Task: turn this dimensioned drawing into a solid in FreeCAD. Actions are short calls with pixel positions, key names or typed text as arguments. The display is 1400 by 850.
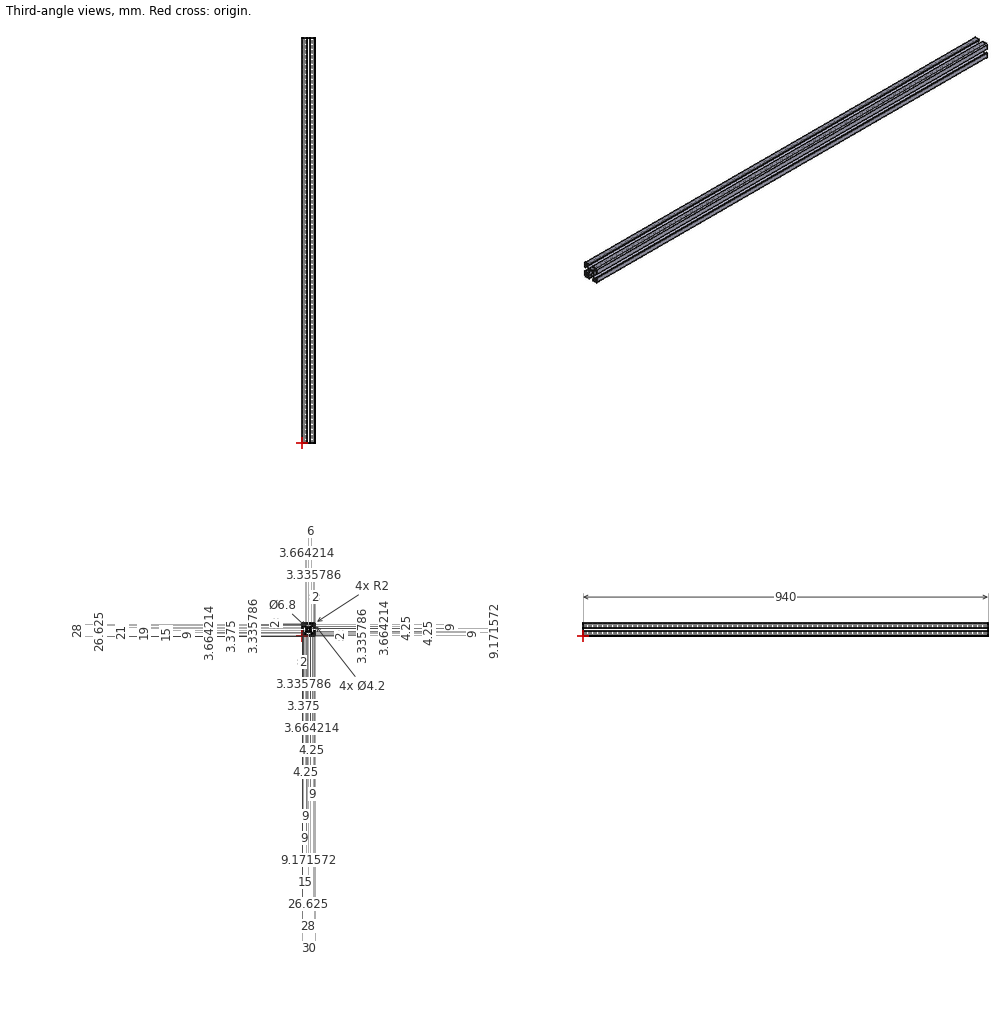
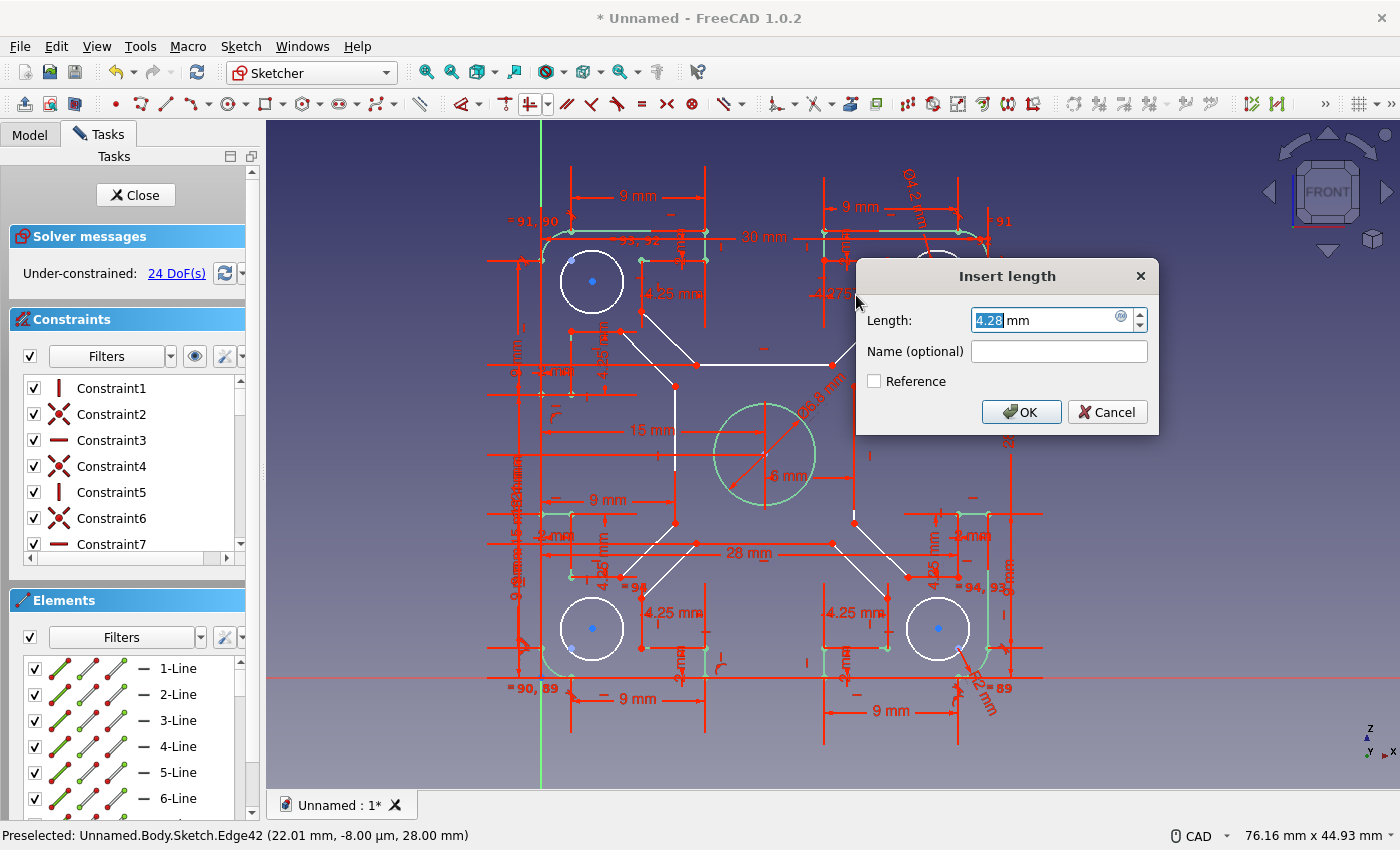
text(4.25)
key(Return)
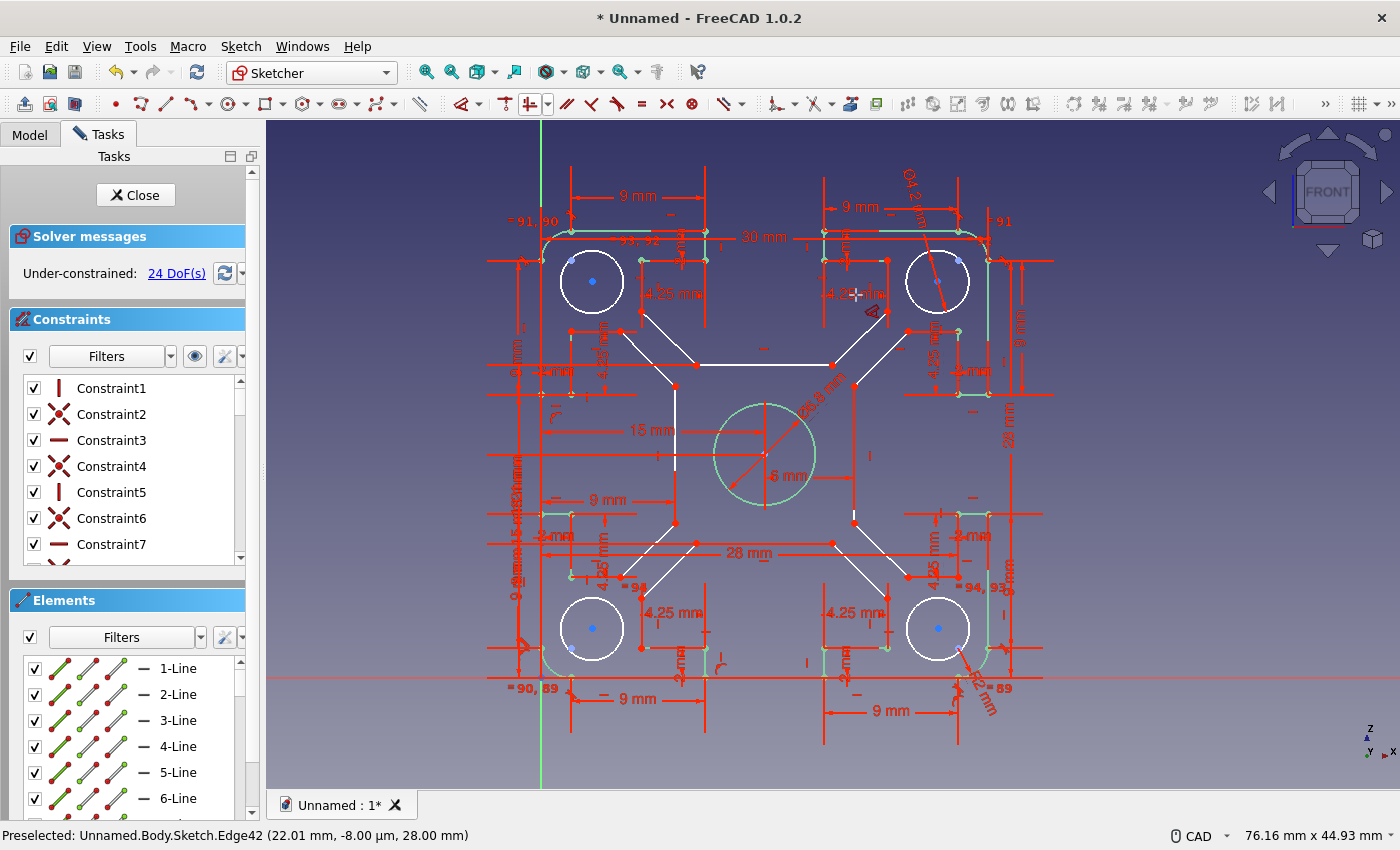
click(592, 282)
click(567, 712)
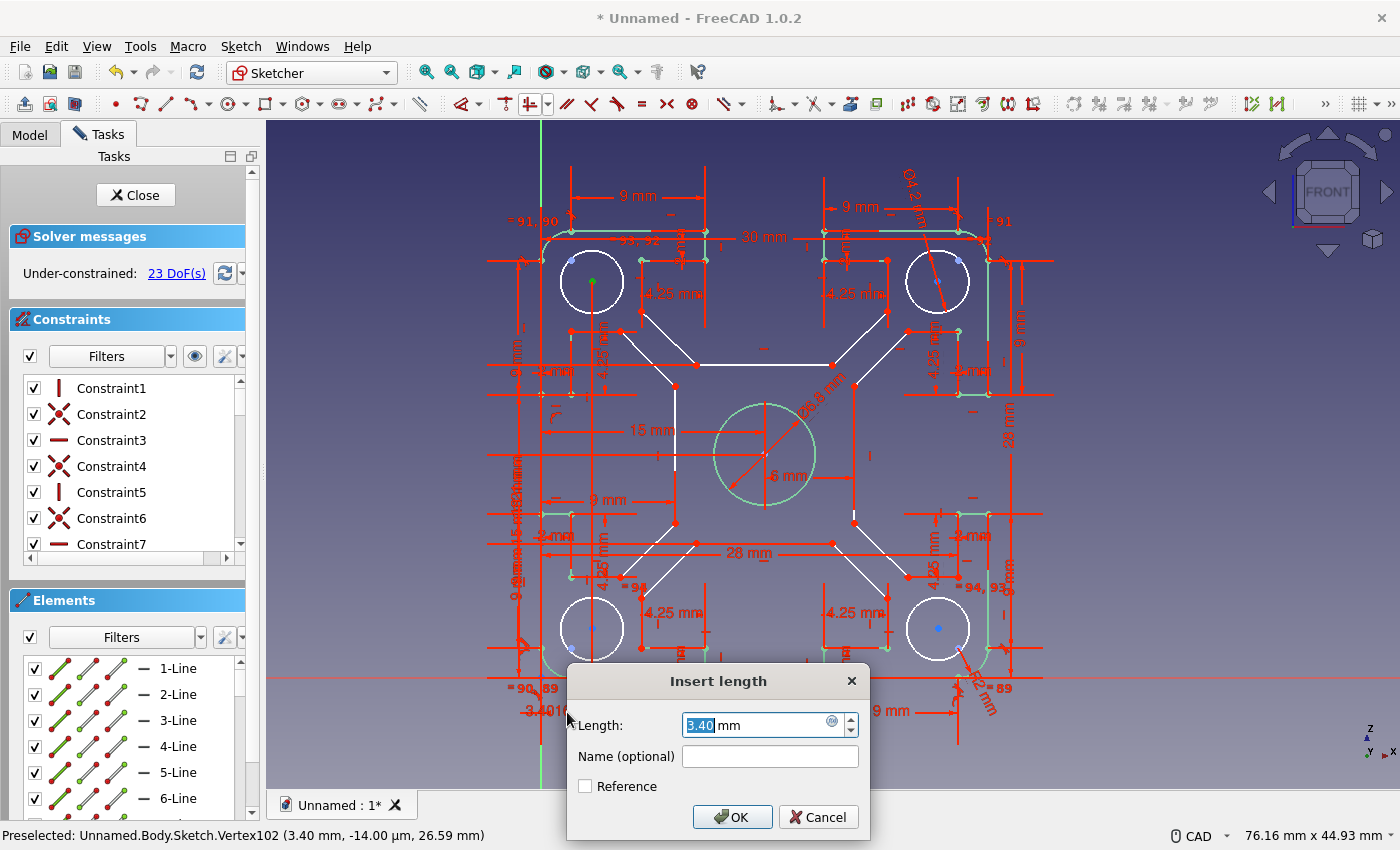
text(3.375)
key(Return)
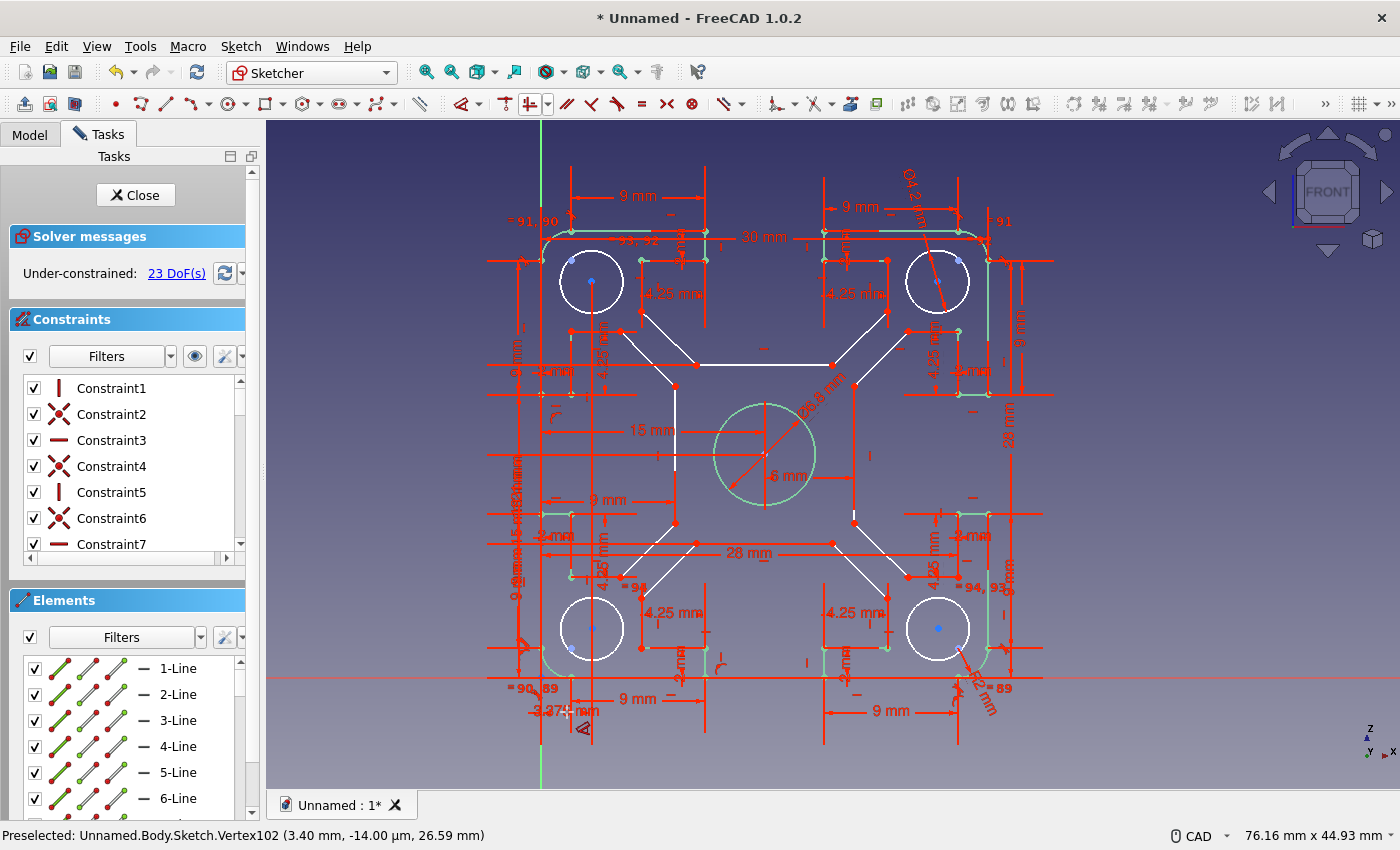
click(938, 629)
click(507, 653)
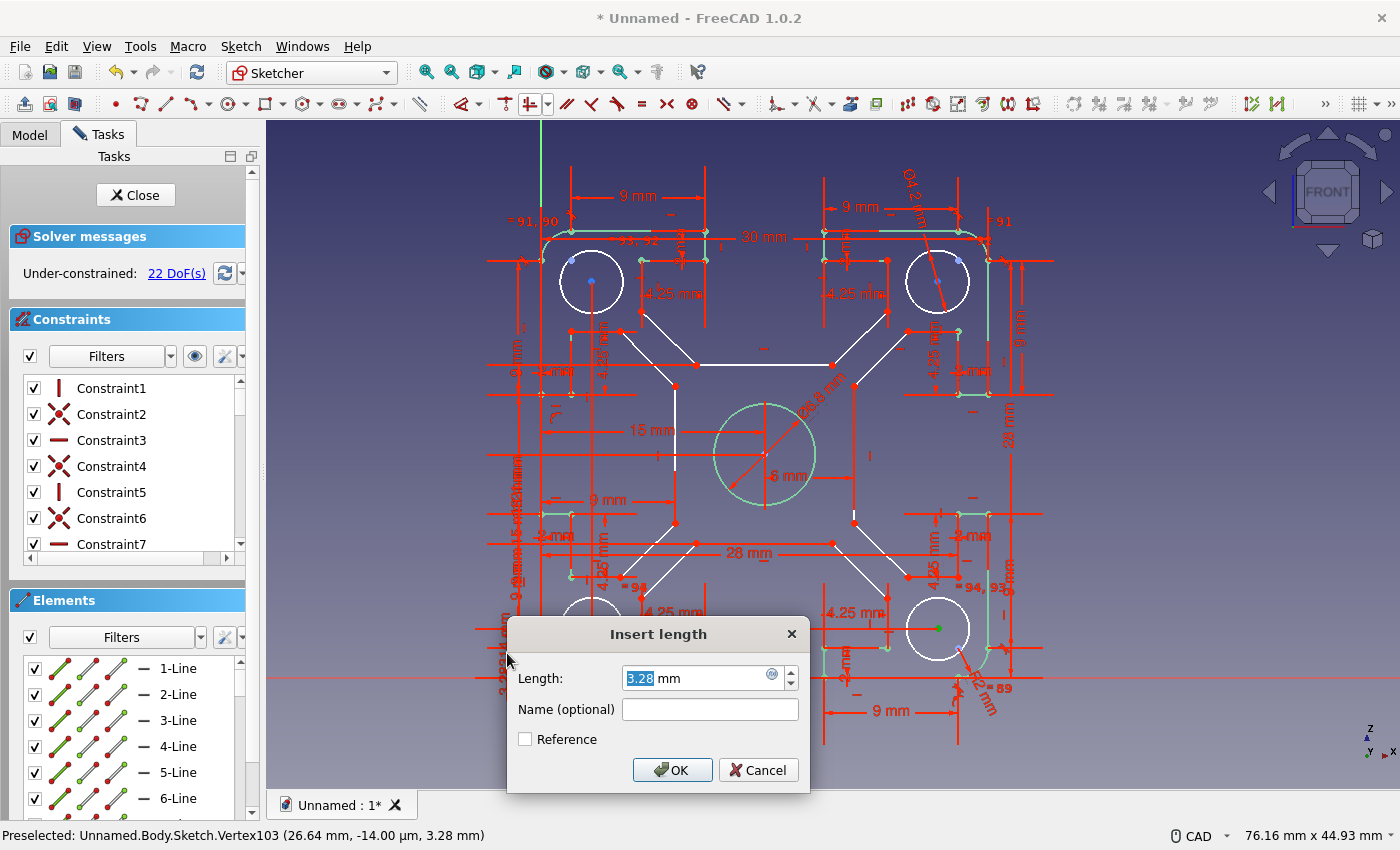
text(3.375)
key(Return)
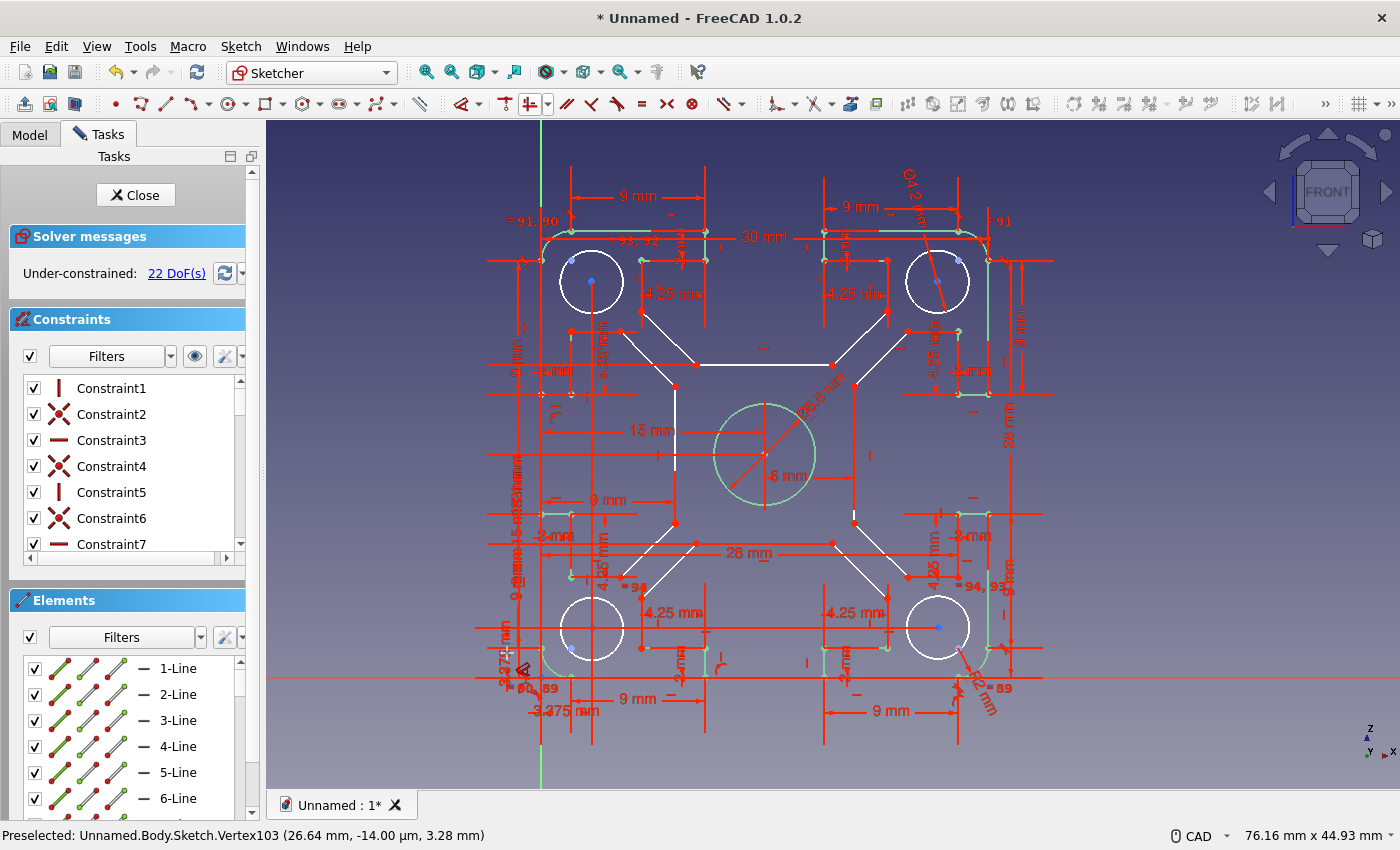
click(592, 629)
click(567, 736)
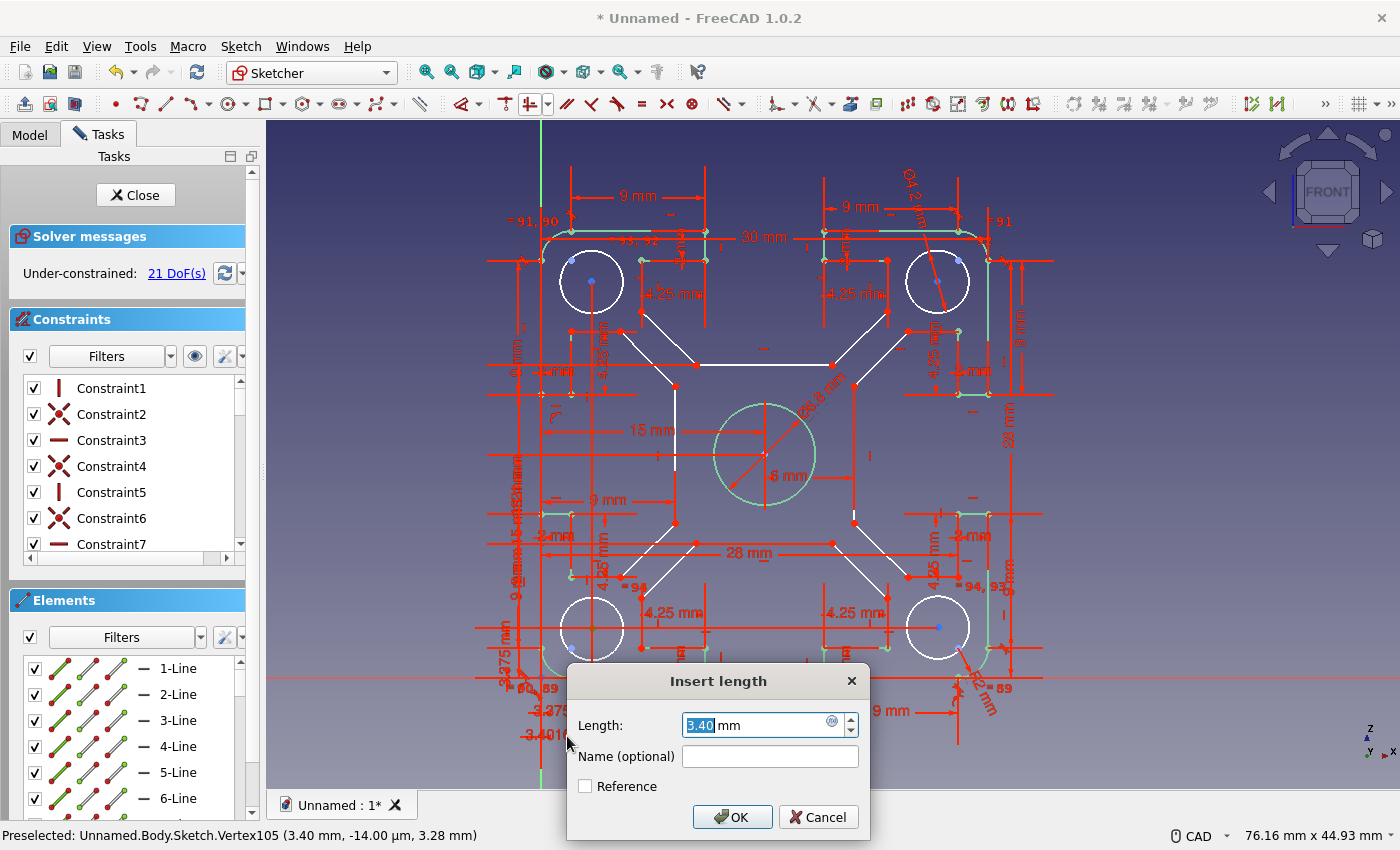
text(3.375)
key(Return)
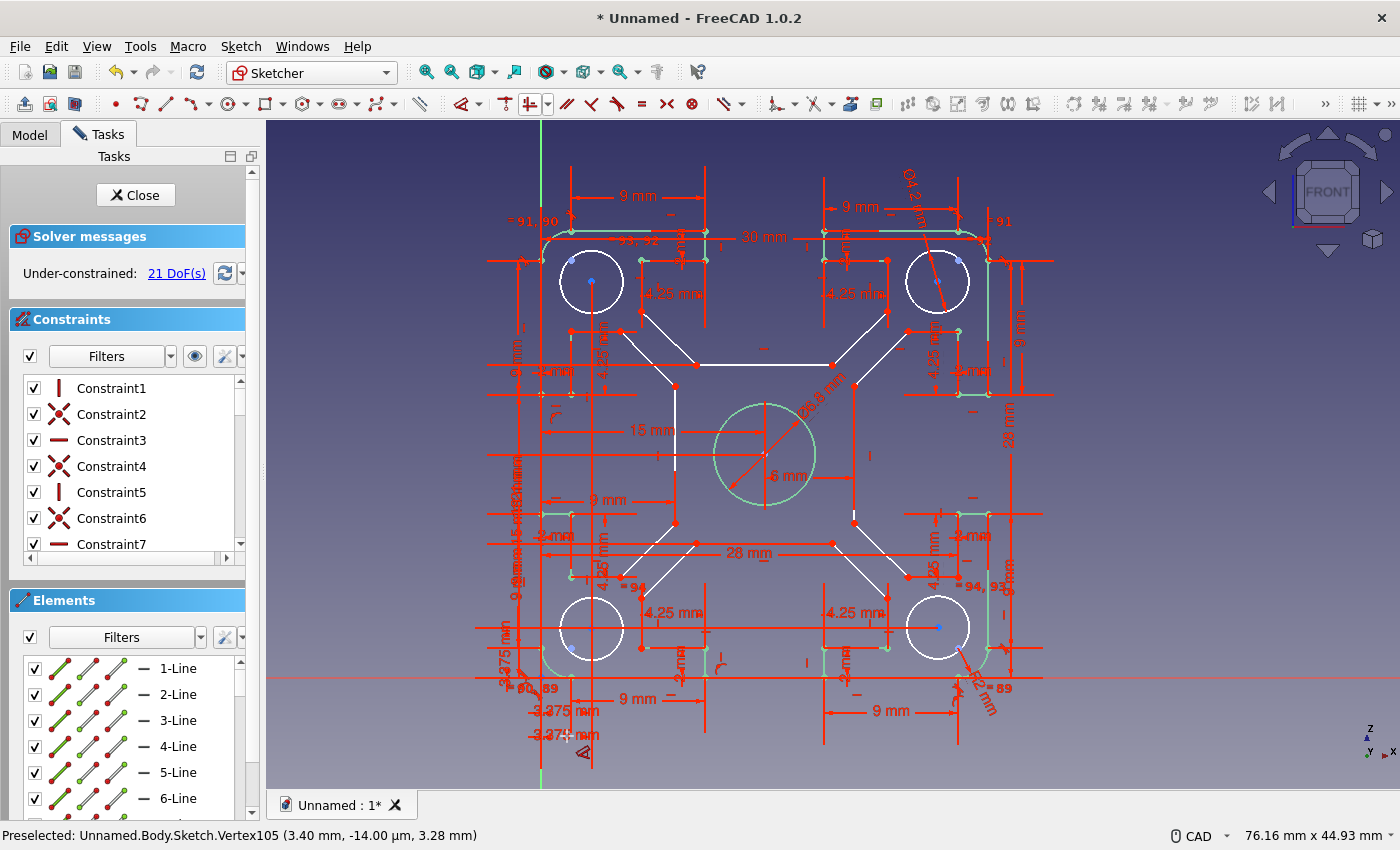
click(592, 629)
click(435, 653)